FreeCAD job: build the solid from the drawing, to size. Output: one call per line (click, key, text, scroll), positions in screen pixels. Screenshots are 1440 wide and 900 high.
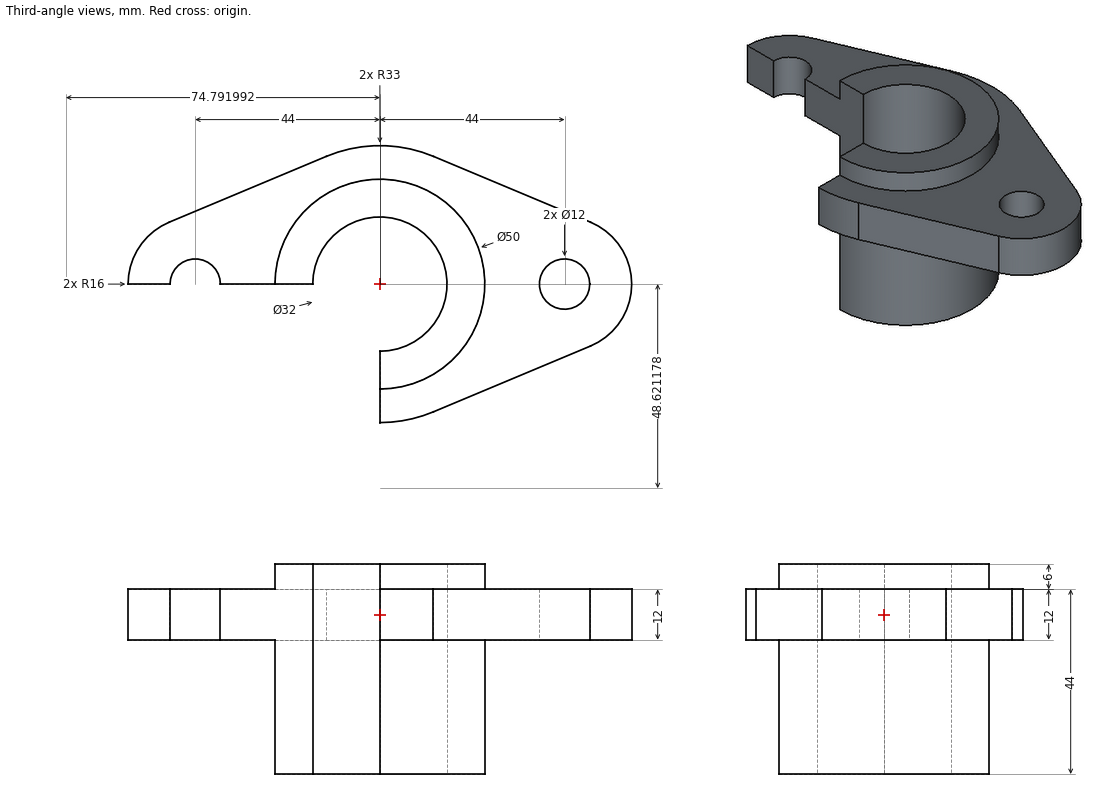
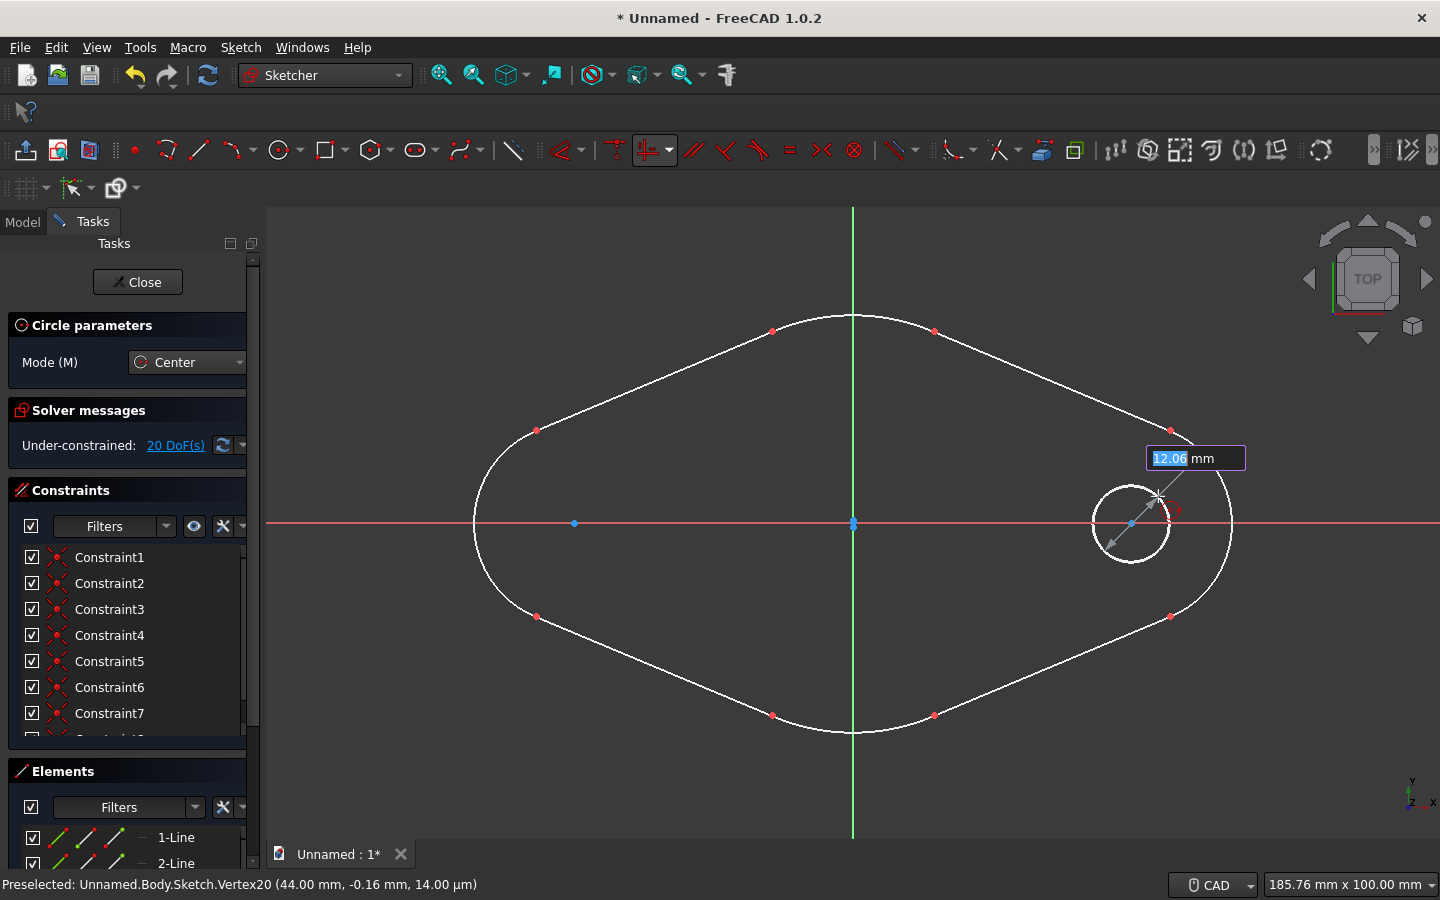
text(12)
key(Return)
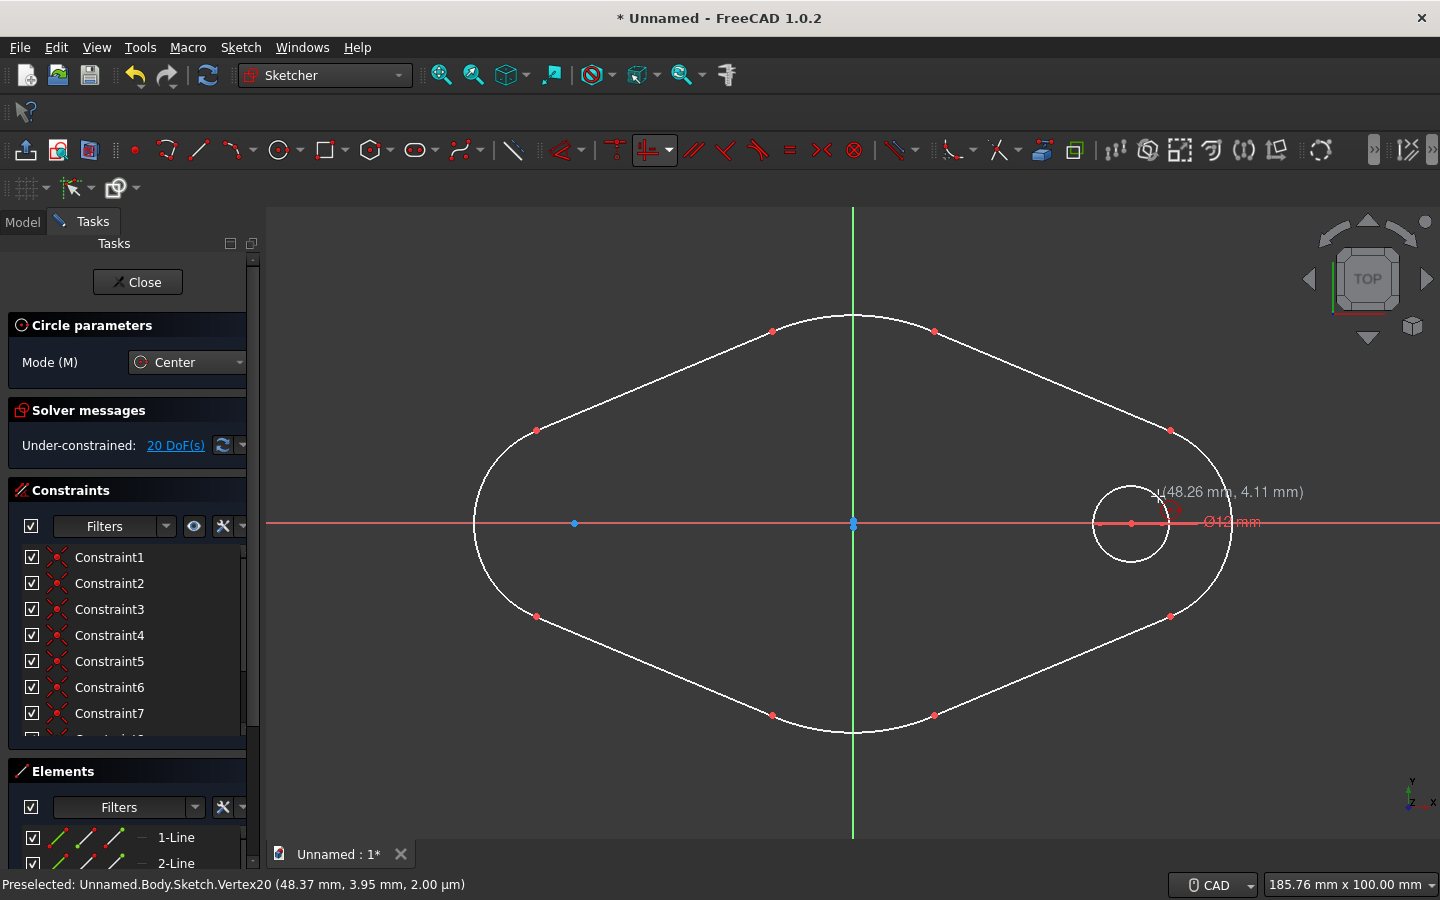
click(575, 523)
move(602, 496)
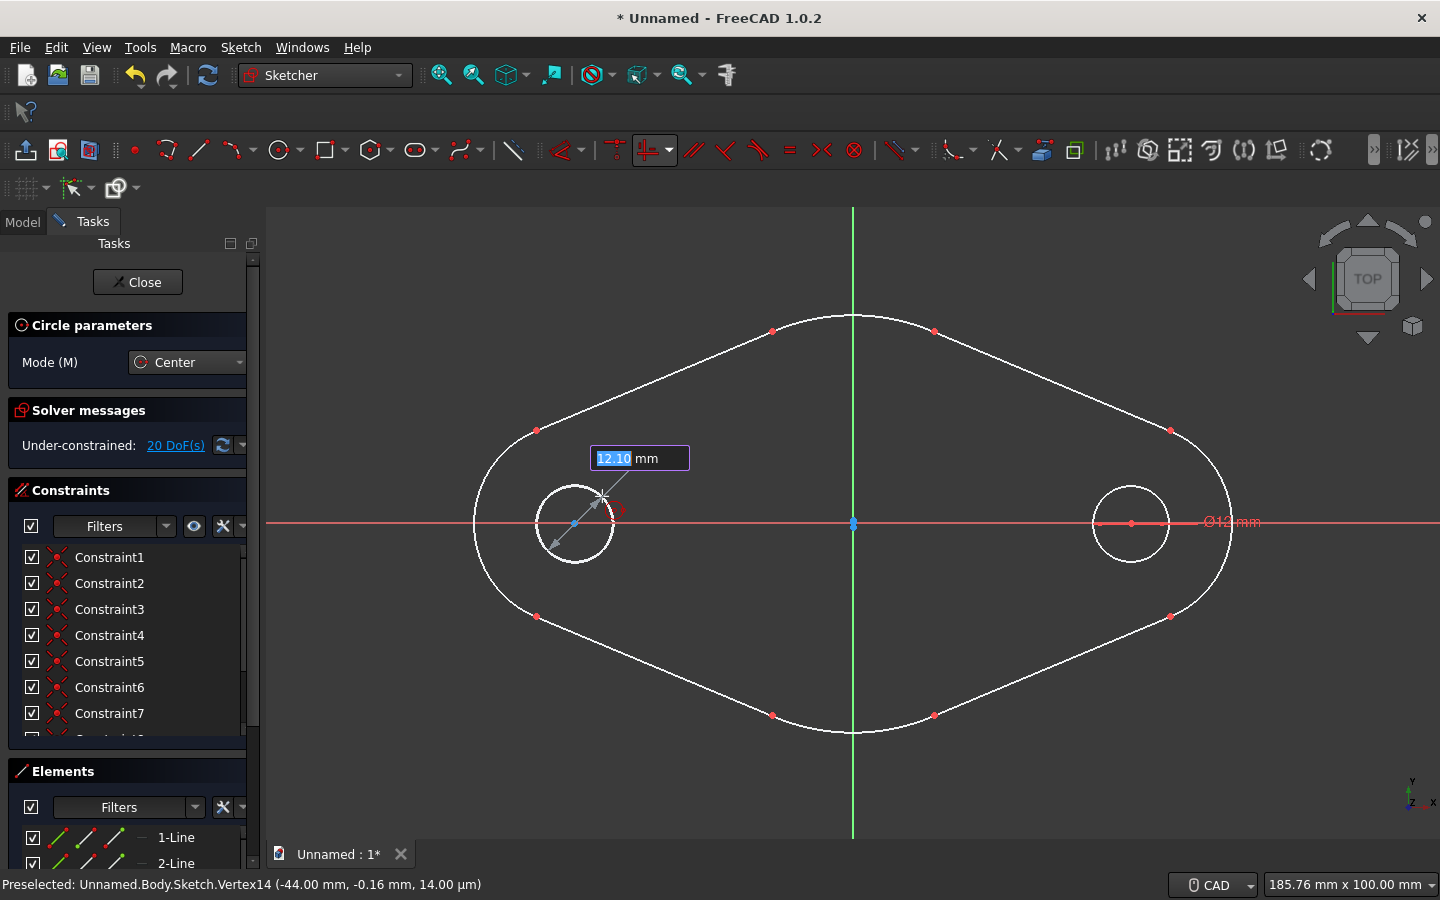
text(12)
key(Return)
key(Escape)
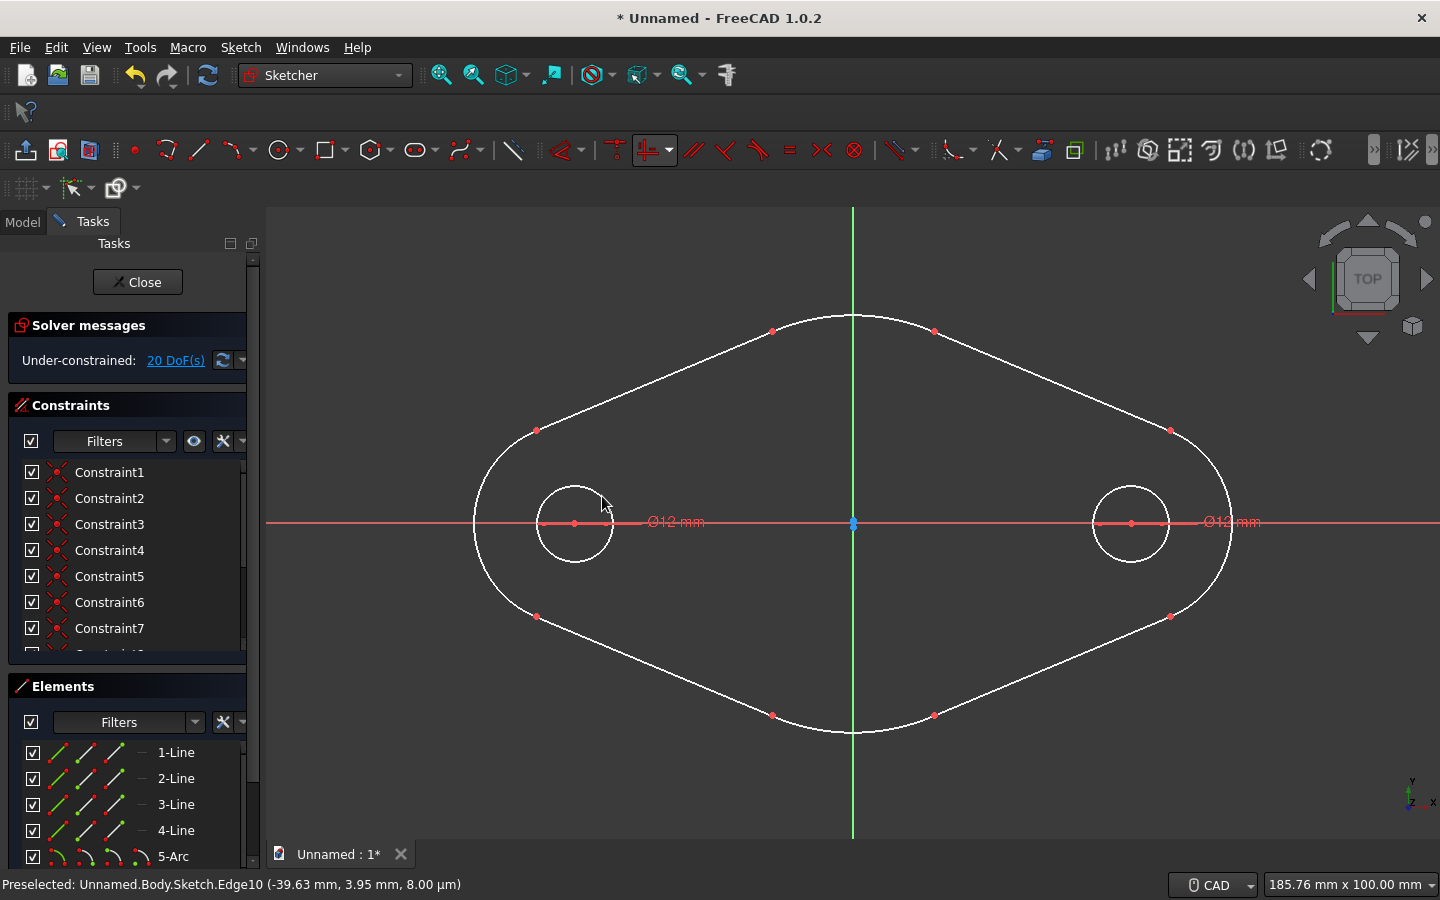
click(1099, 401)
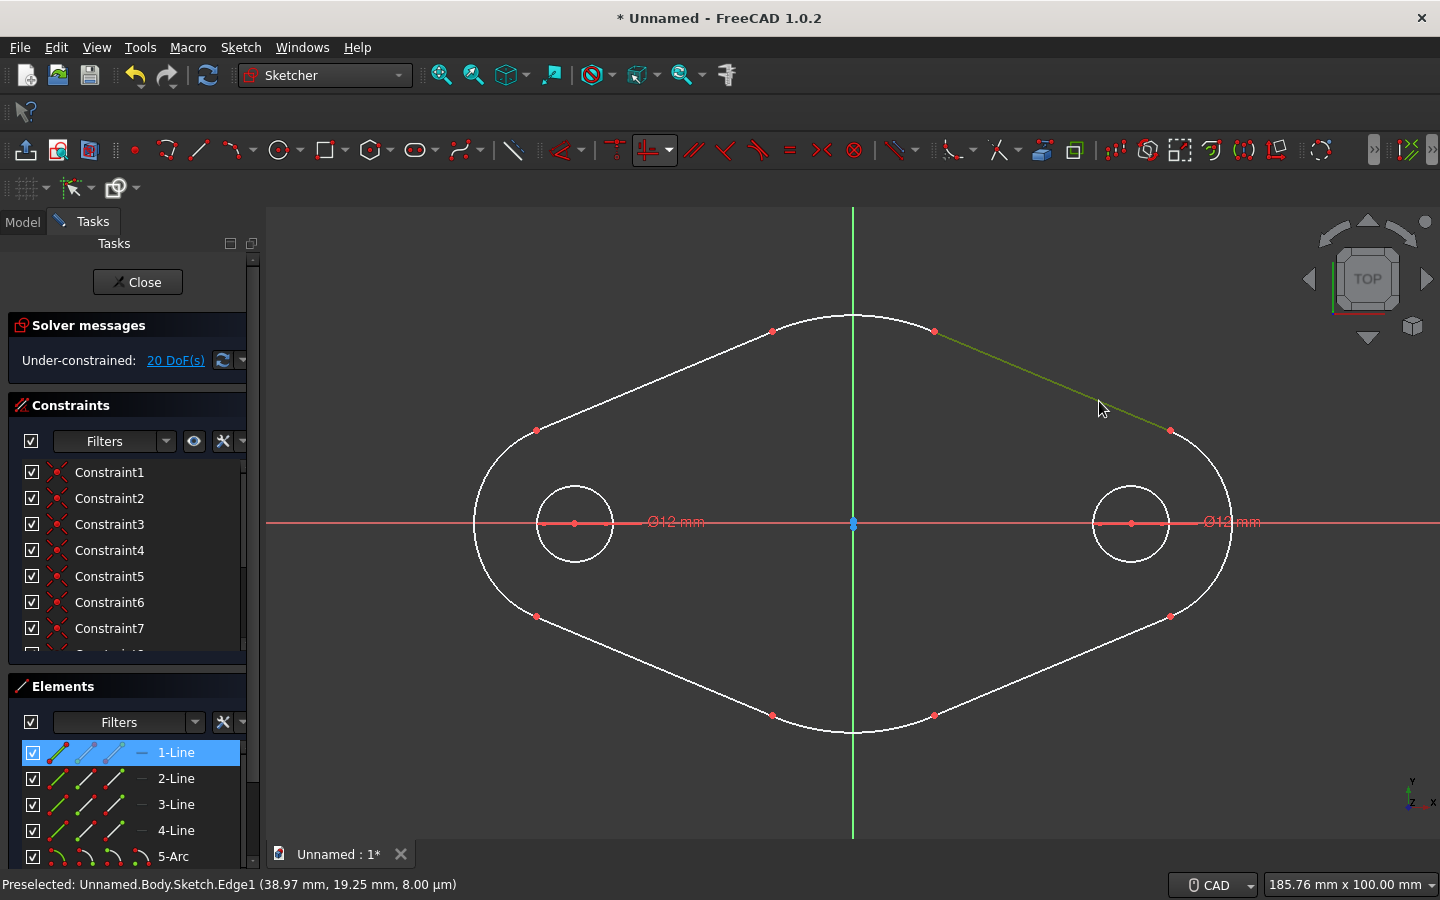
click(886, 318)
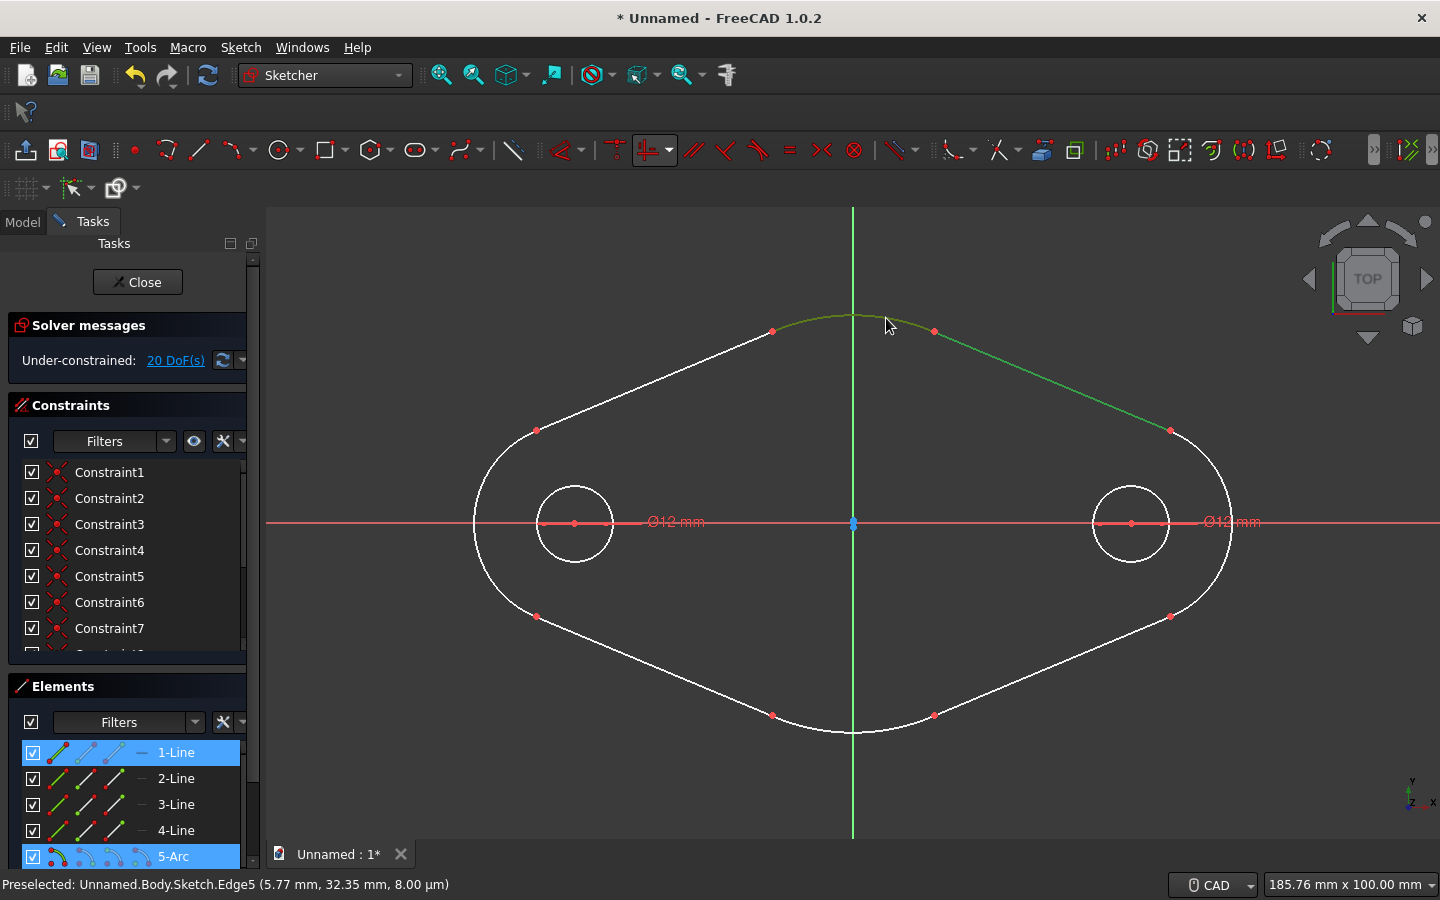
click(758, 150)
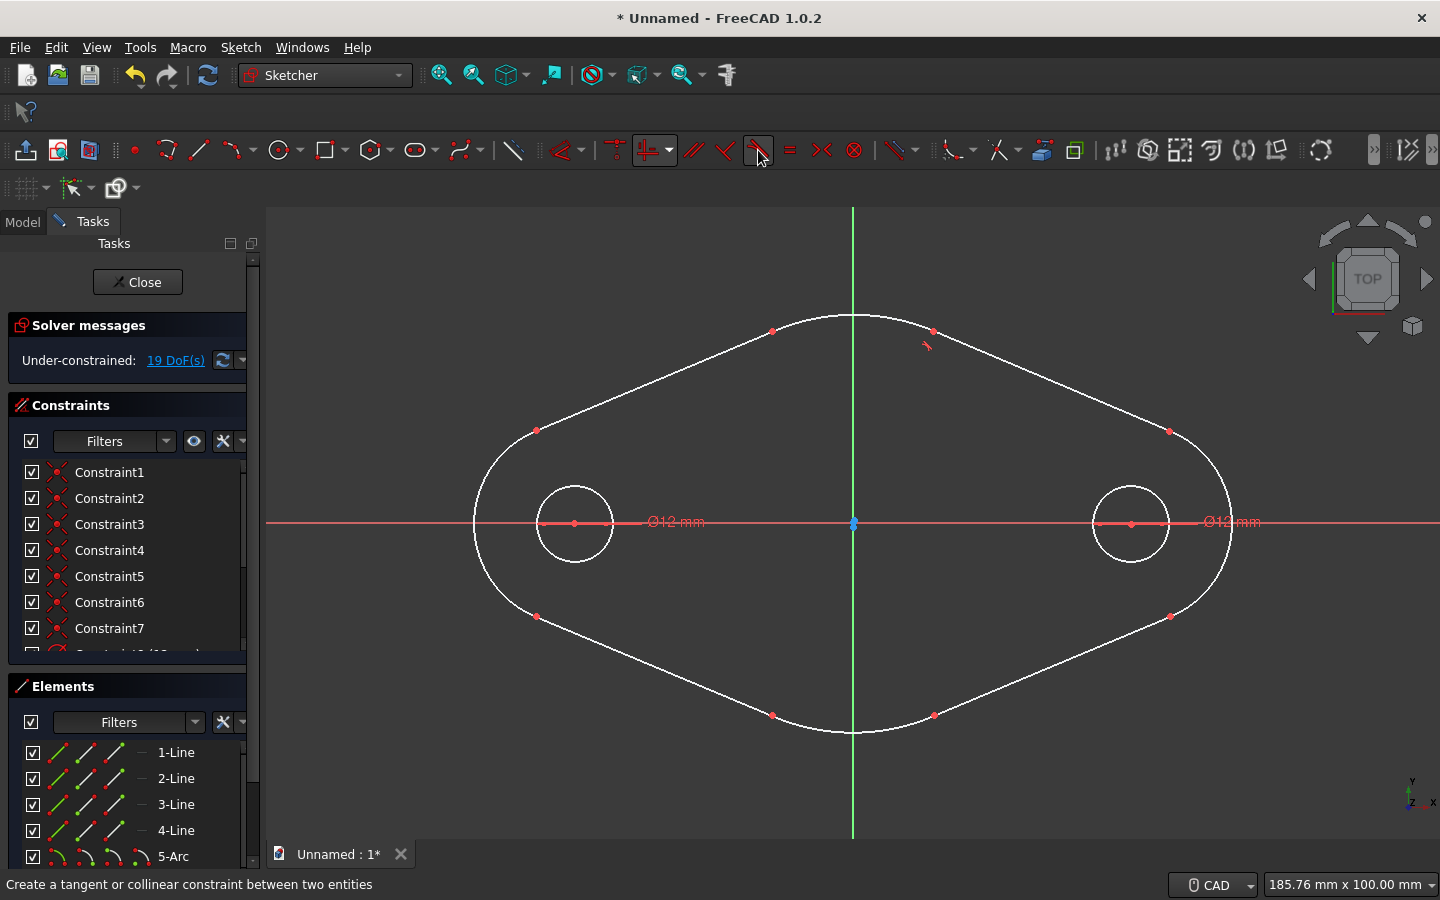
click(1099, 401)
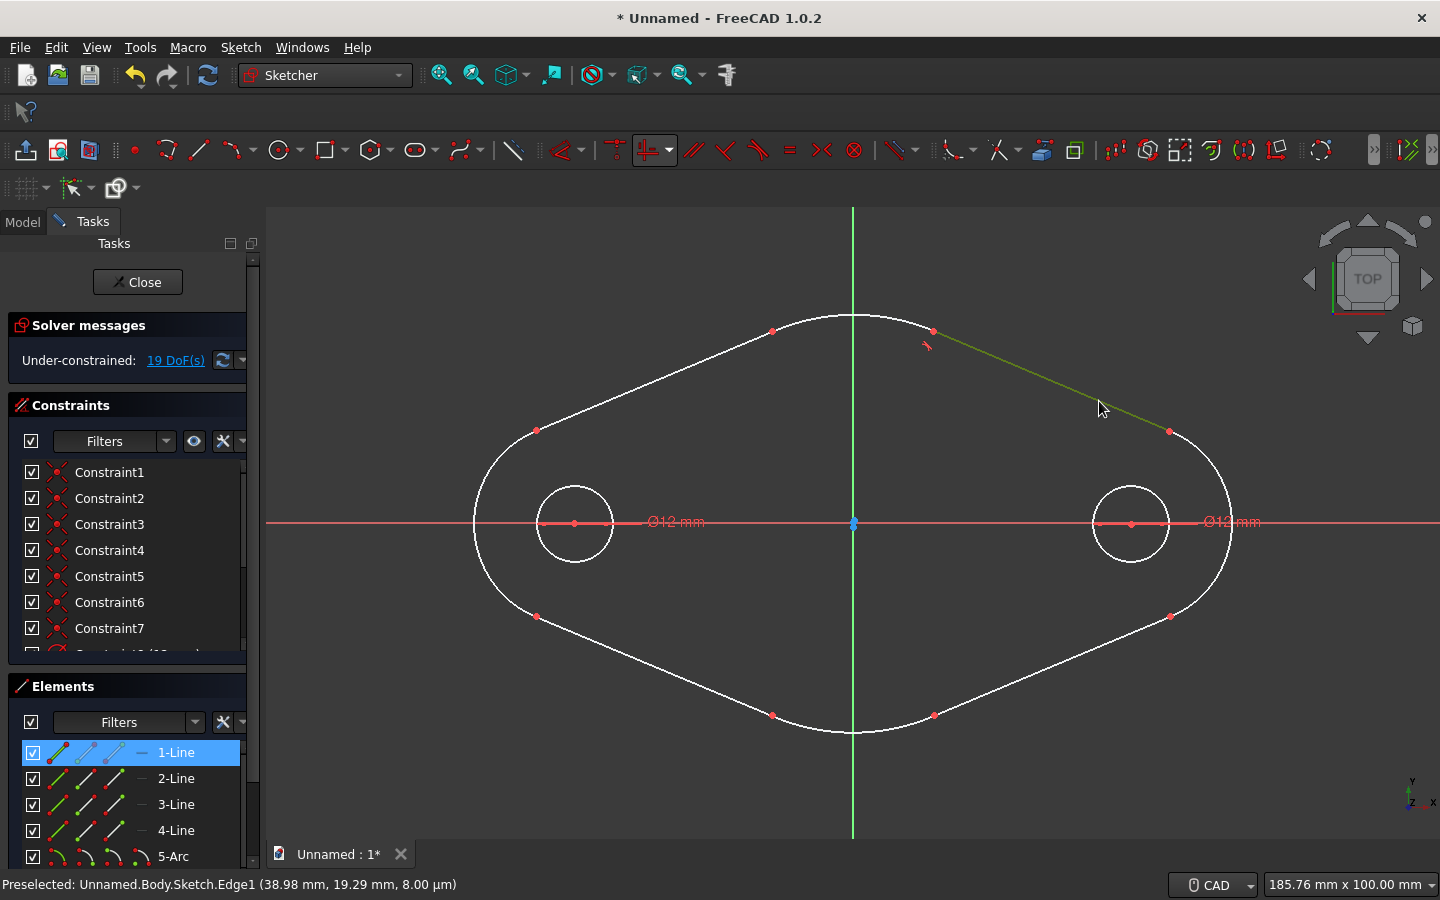
click(1221, 570)